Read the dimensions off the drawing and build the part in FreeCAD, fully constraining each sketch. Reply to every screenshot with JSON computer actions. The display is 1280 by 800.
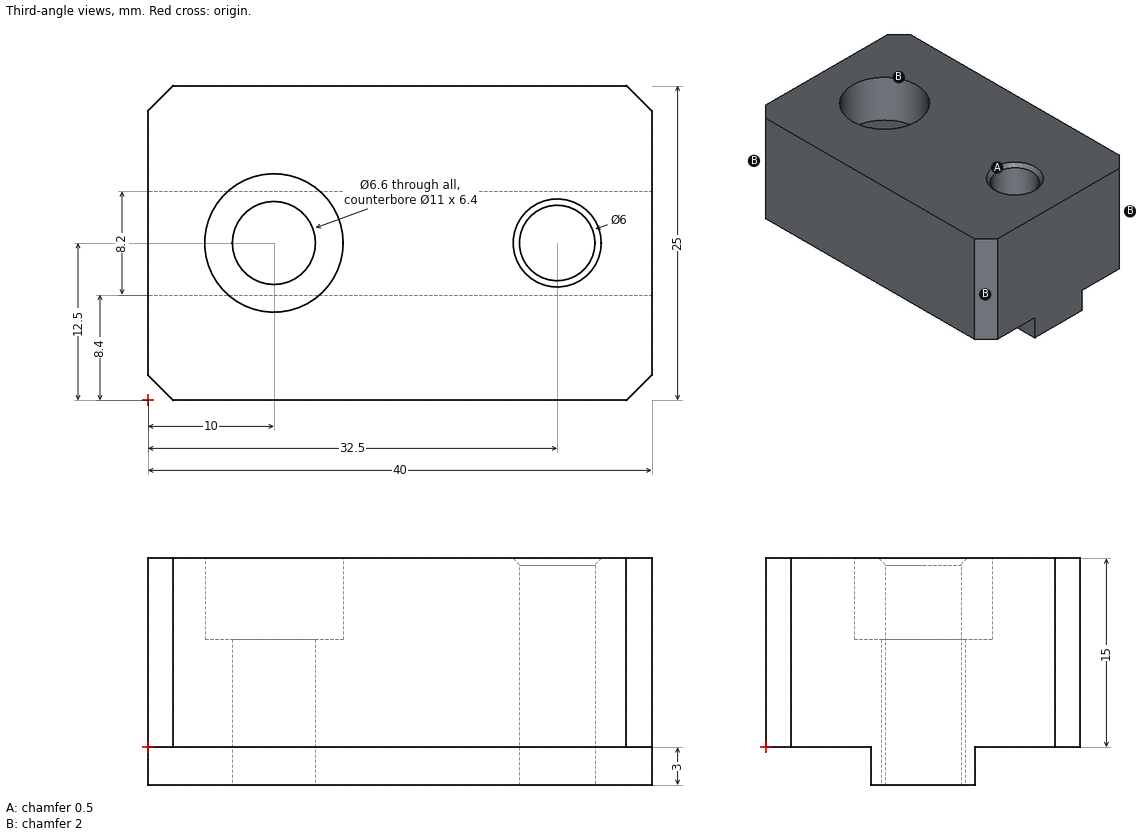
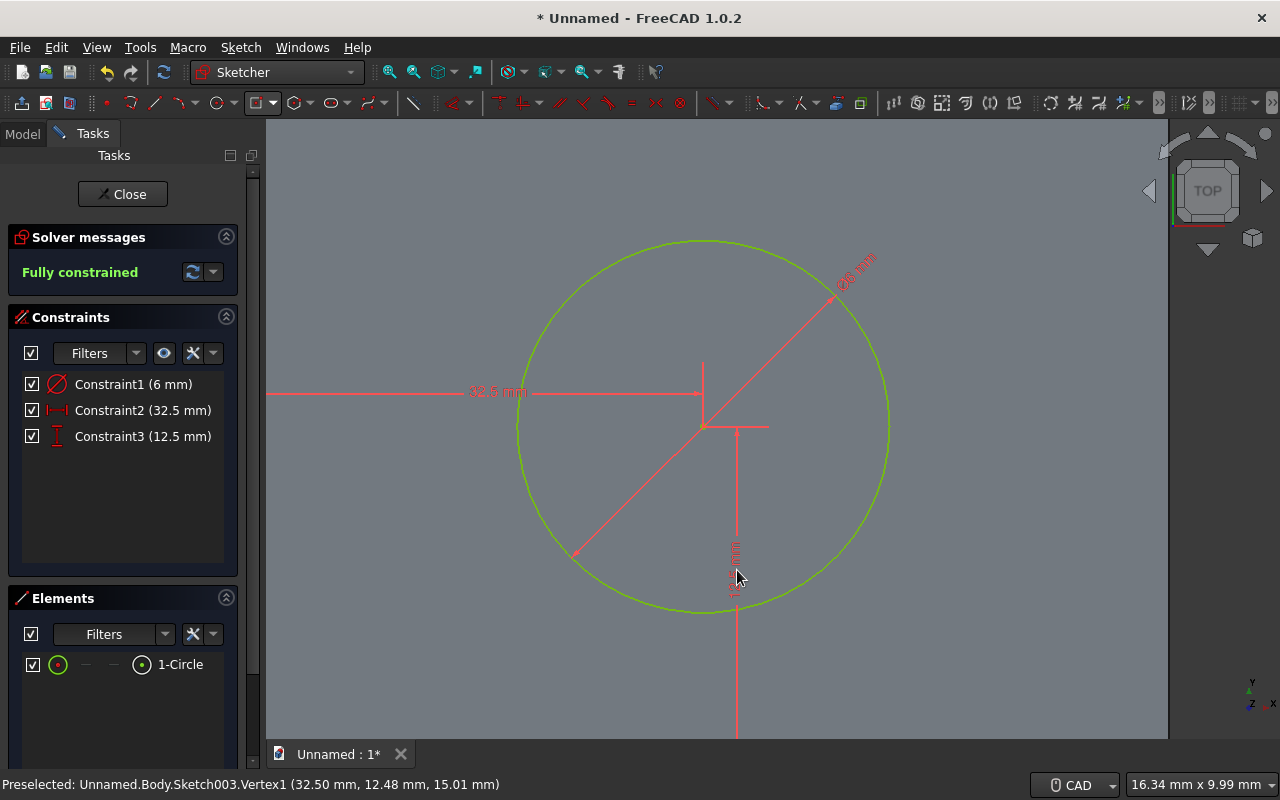
{"action": "left_click", "coordinate": [123, 194]}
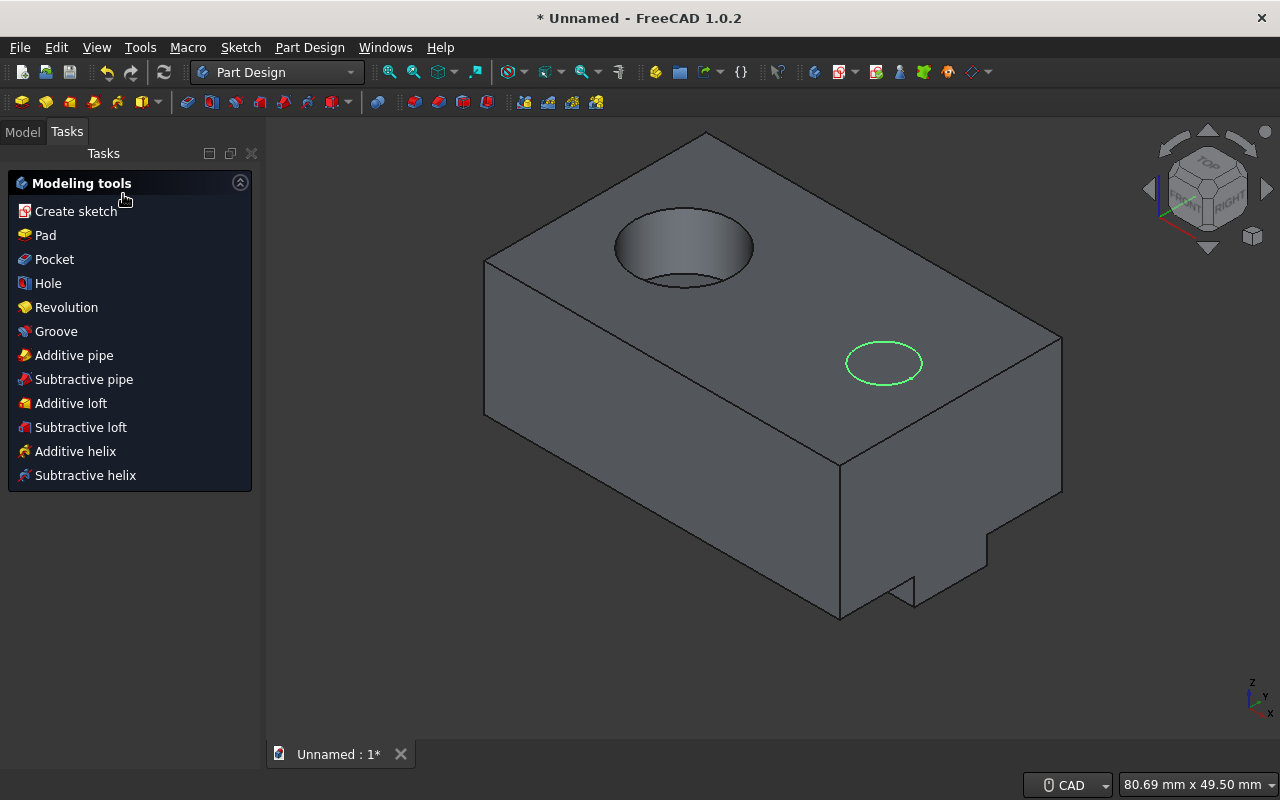
{"action": "left_click", "coordinate": [188, 102]}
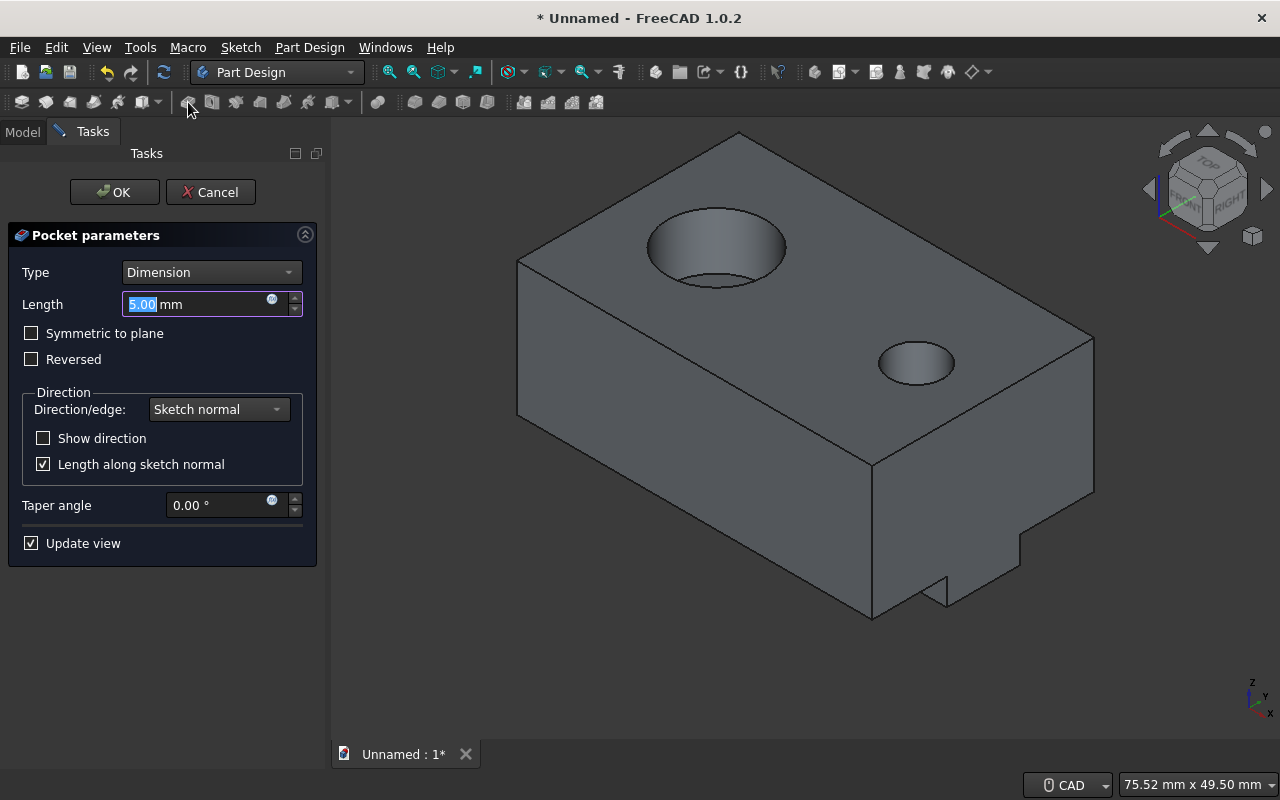
{"action": "left_click", "coordinate": [212, 272]}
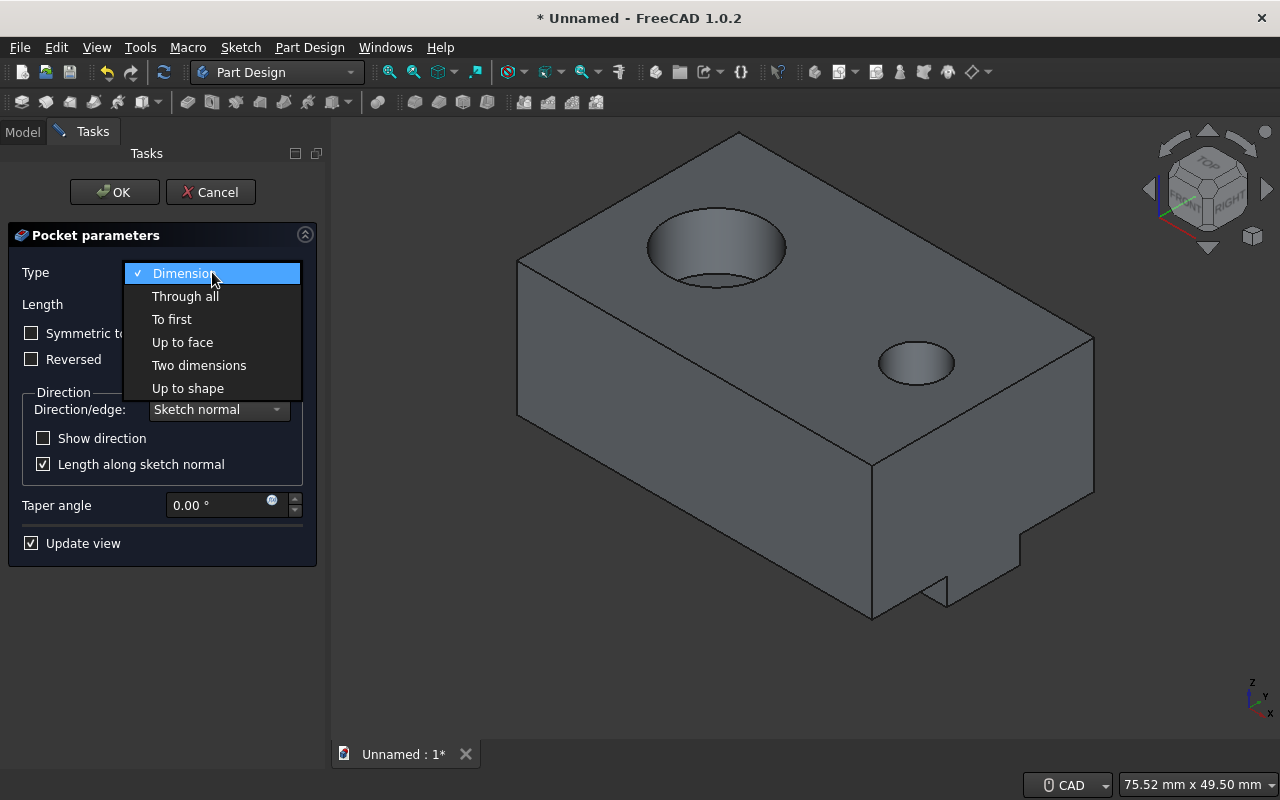
{"action": "left_click", "coordinate": [212, 296]}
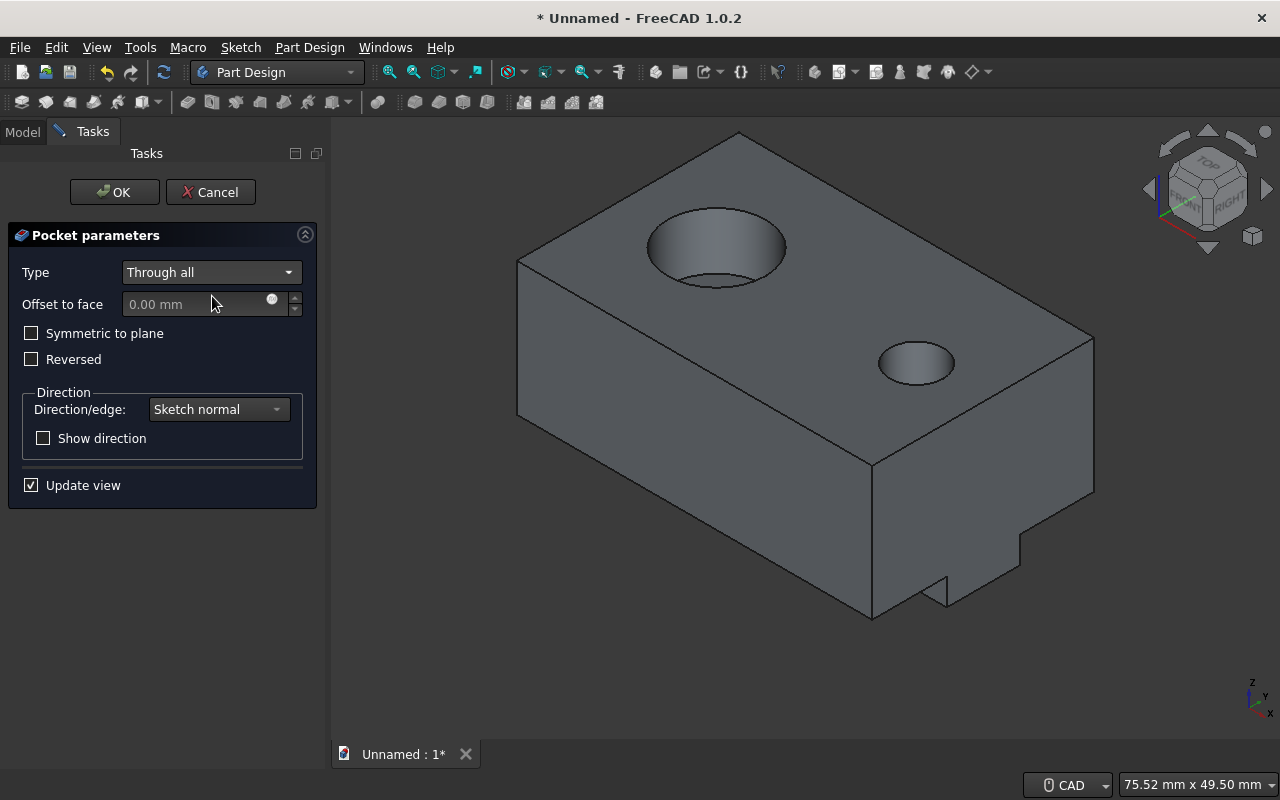
{"action": "left_click", "coordinate": [115, 192]}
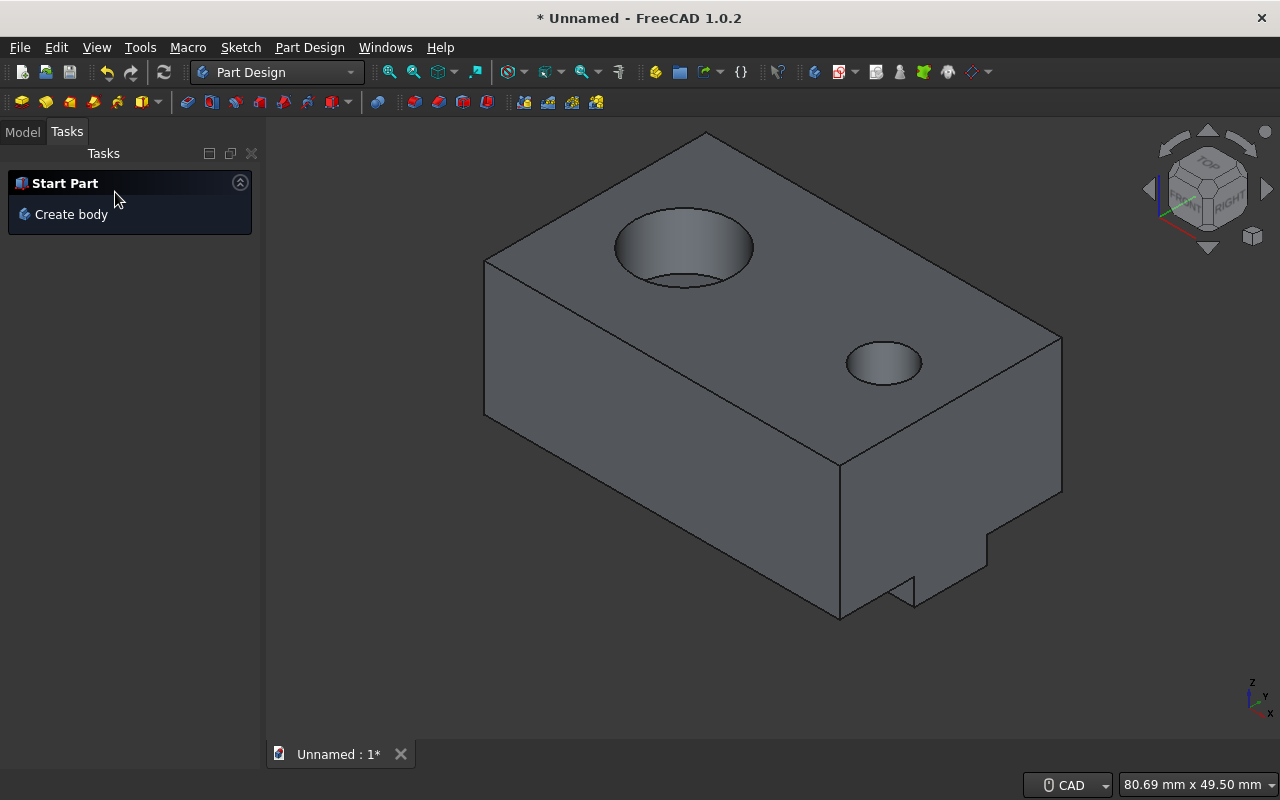
{"action": "left_click", "coordinate": [857, 347]}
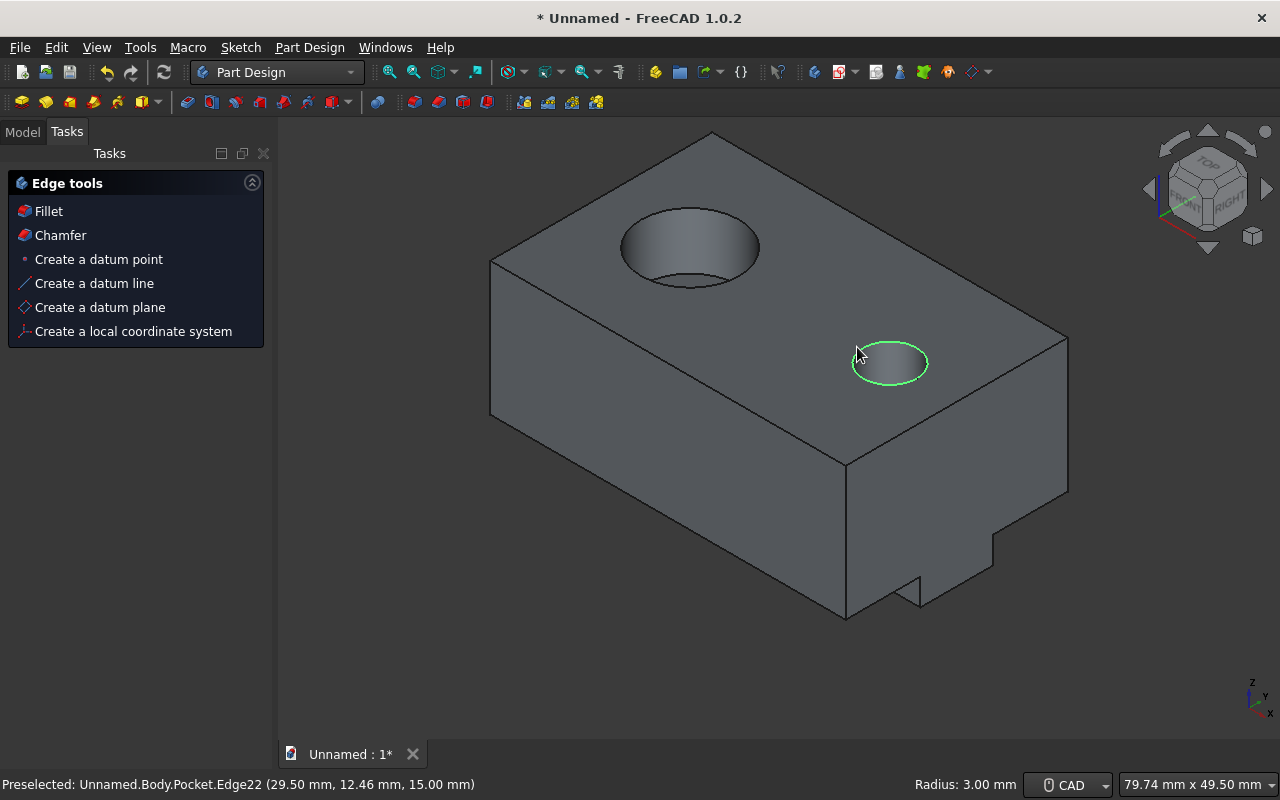
{"action": "left_click", "coordinate": [440, 102]}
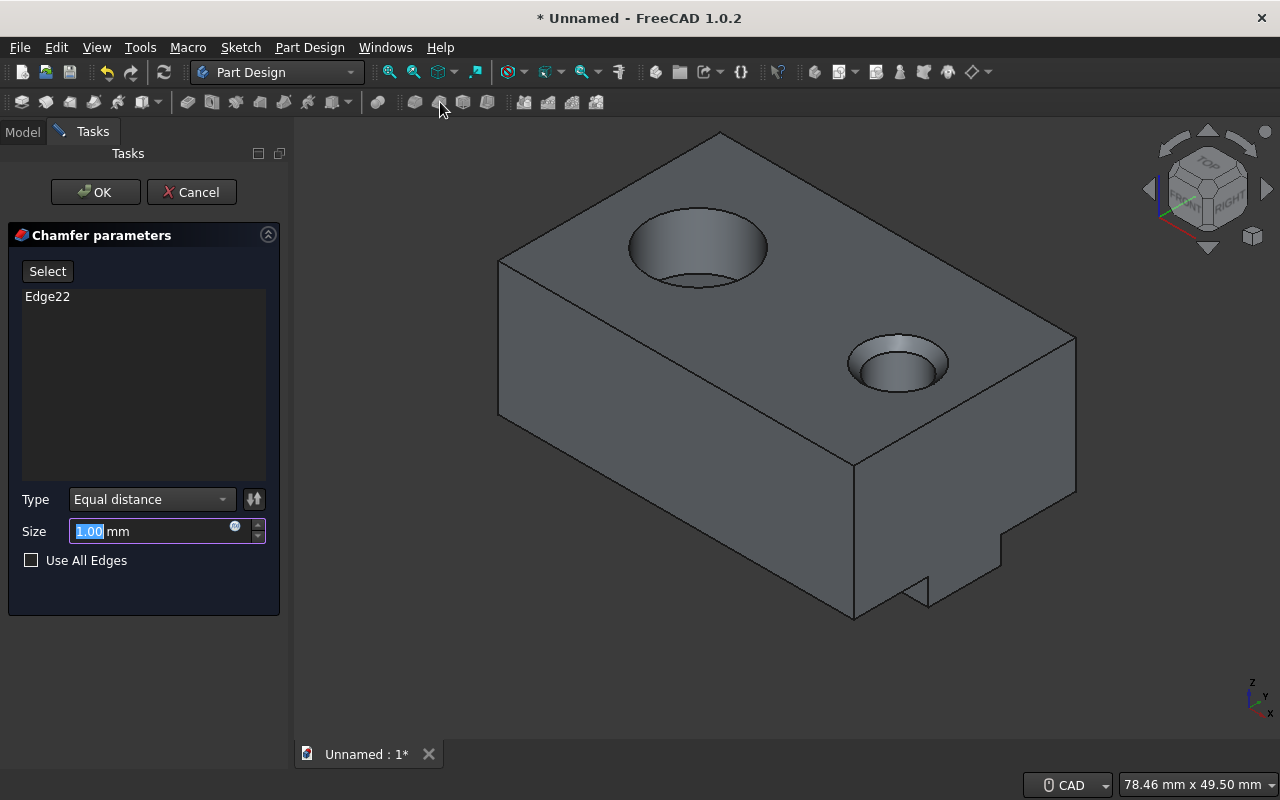
{"action": "type", "text": "0.5"}
{"action": "key", "text": "Tab"}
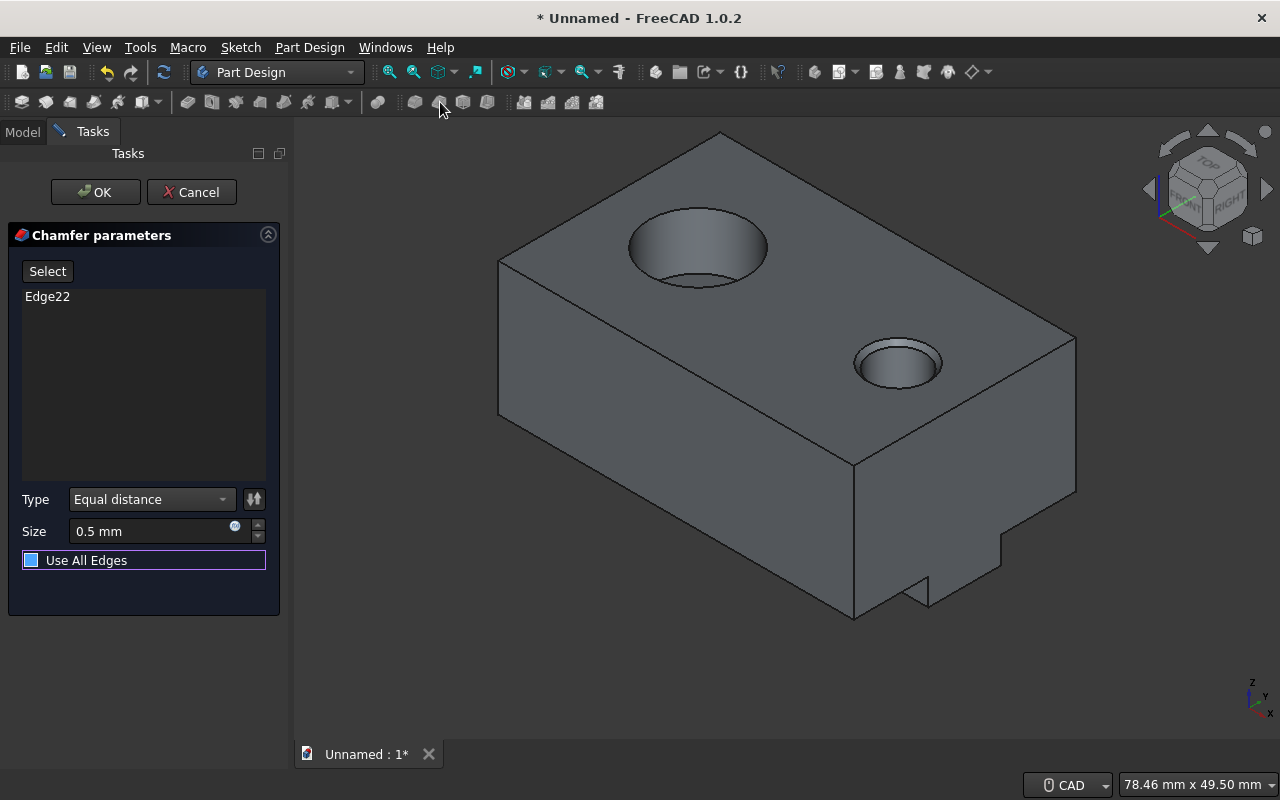
{"action": "left_click", "coordinate": [96, 192]}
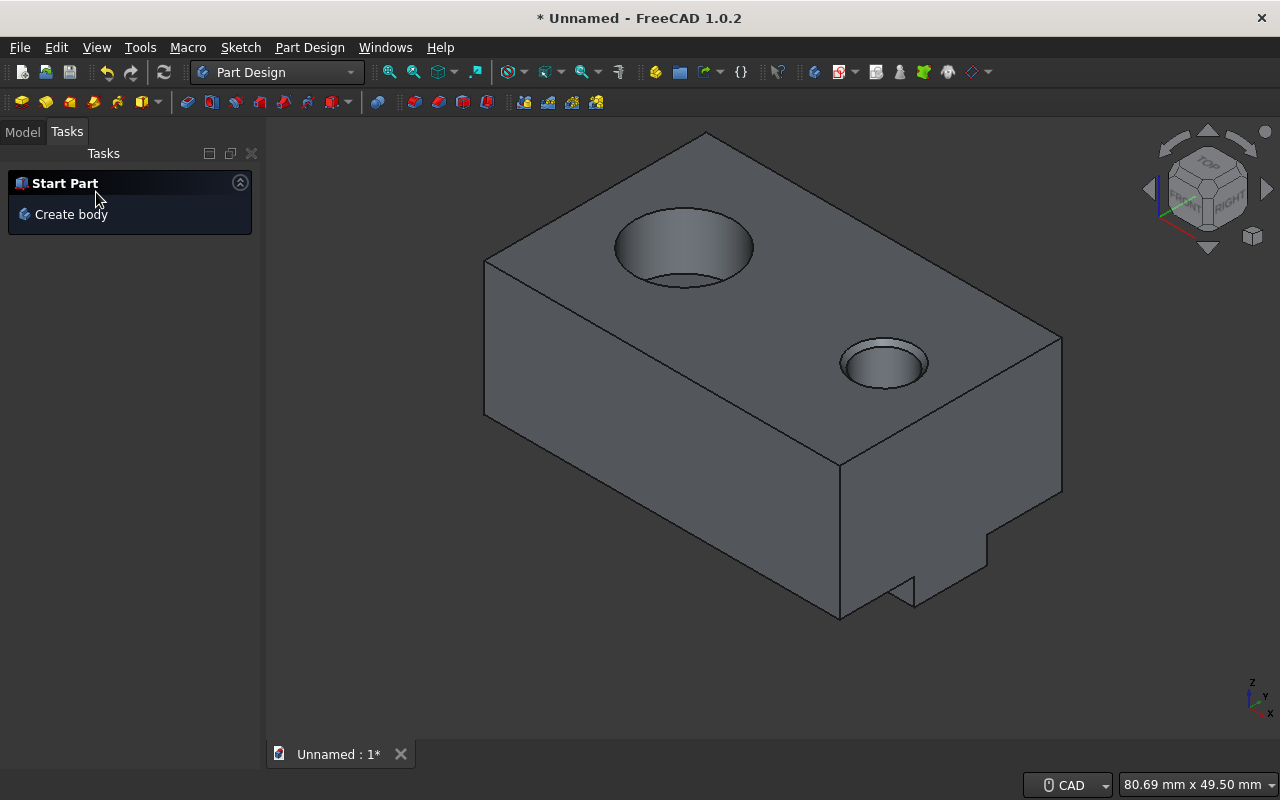
{"action": "left_click", "coordinate": [840, 542]}